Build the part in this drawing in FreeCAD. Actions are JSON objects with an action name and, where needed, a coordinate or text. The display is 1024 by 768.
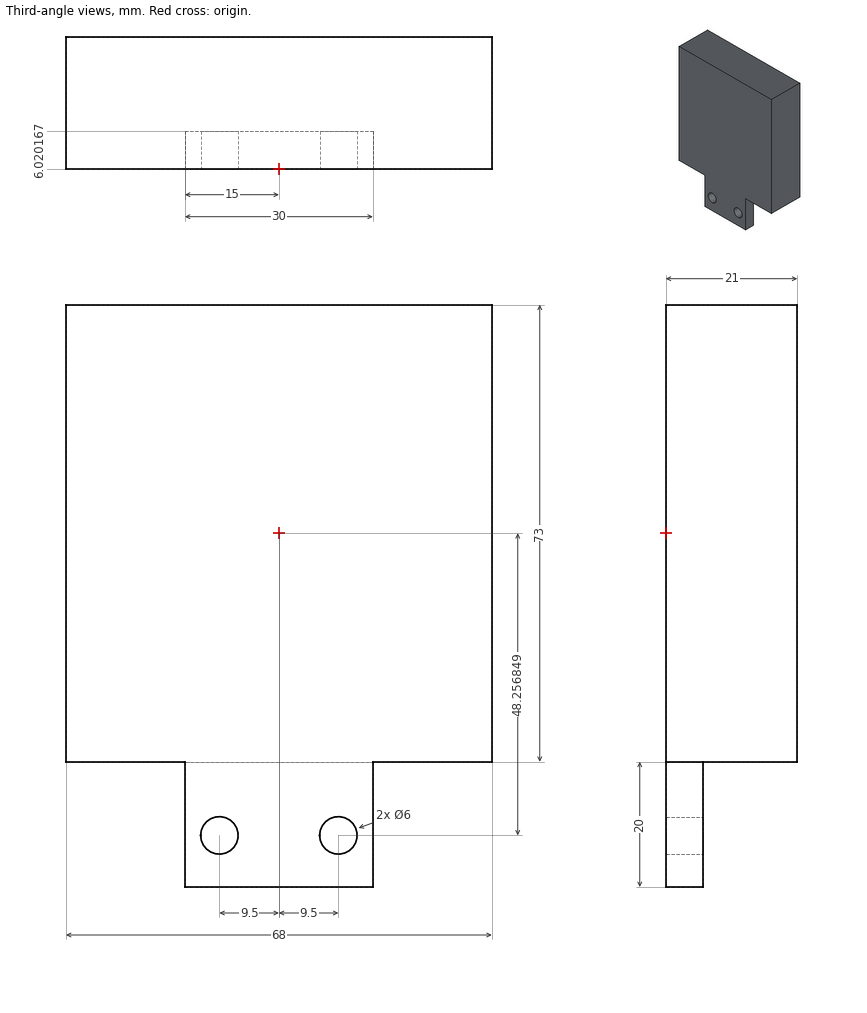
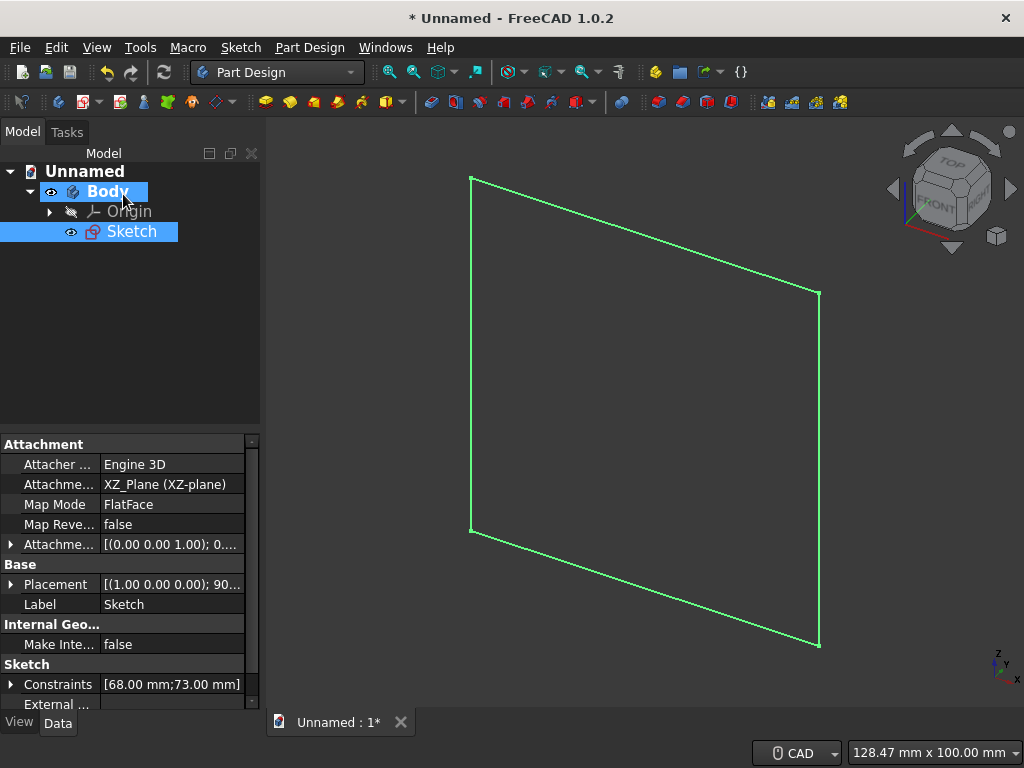
{"action": "left_click", "coordinate": [266, 102]}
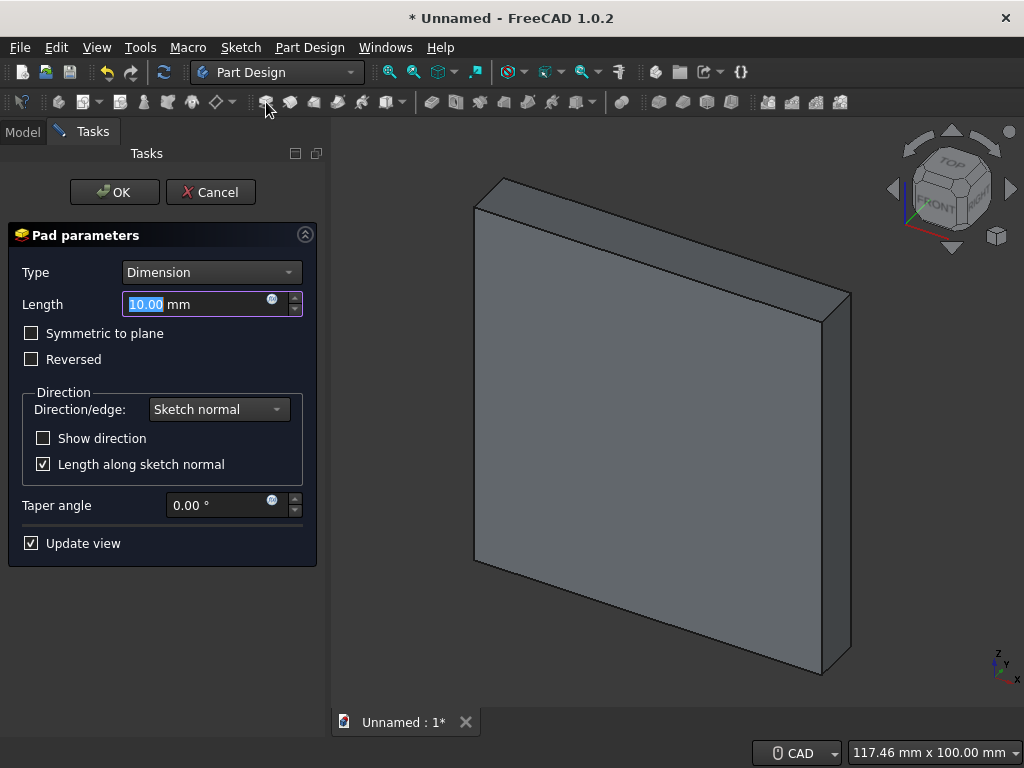
{"action": "type", "text": "21"}
{"action": "key", "text": "Tab"}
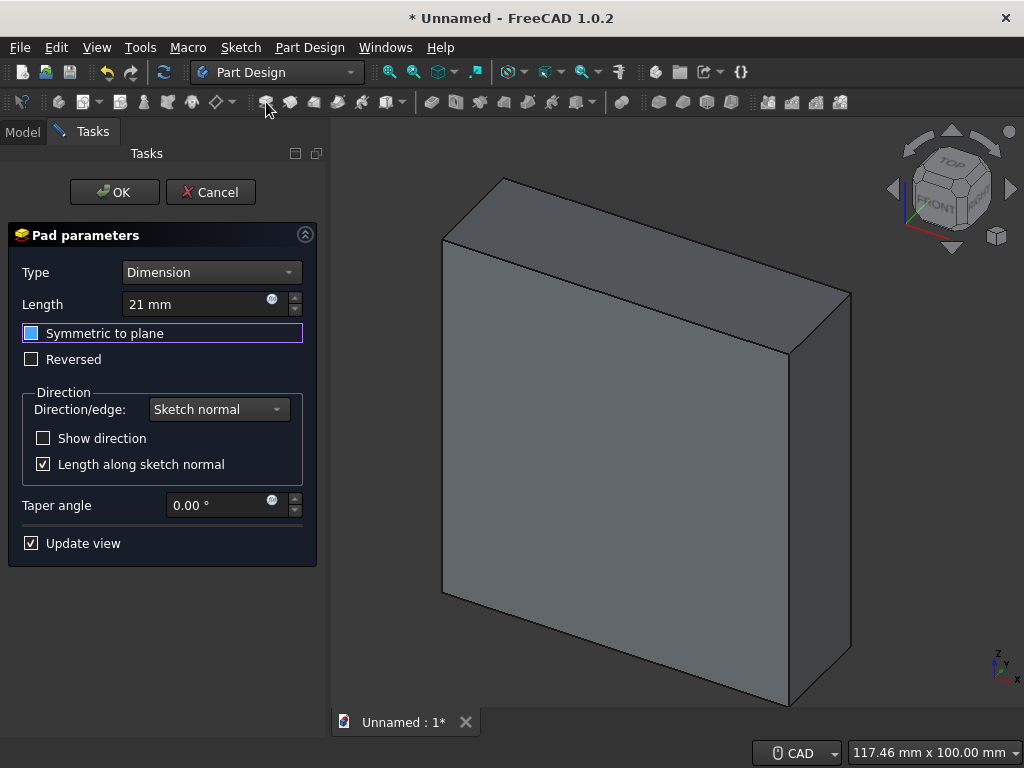
{"action": "left_click", "coordinate": [30, 359]}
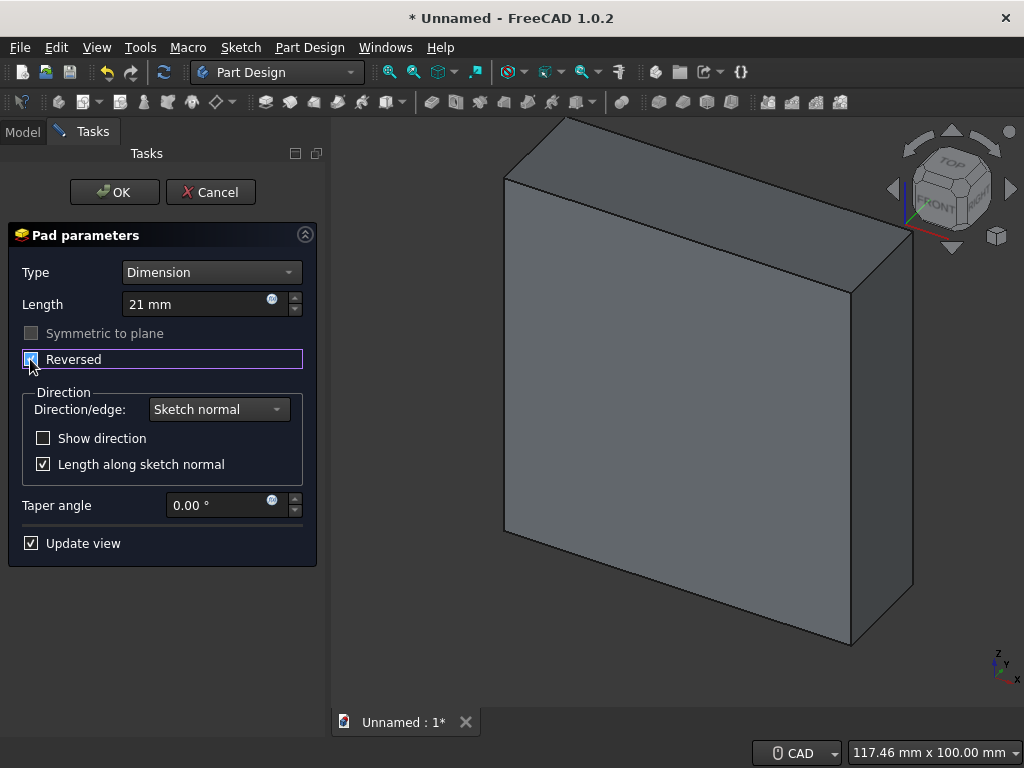
{"action": "left_click", "coordinate": [115, 192]}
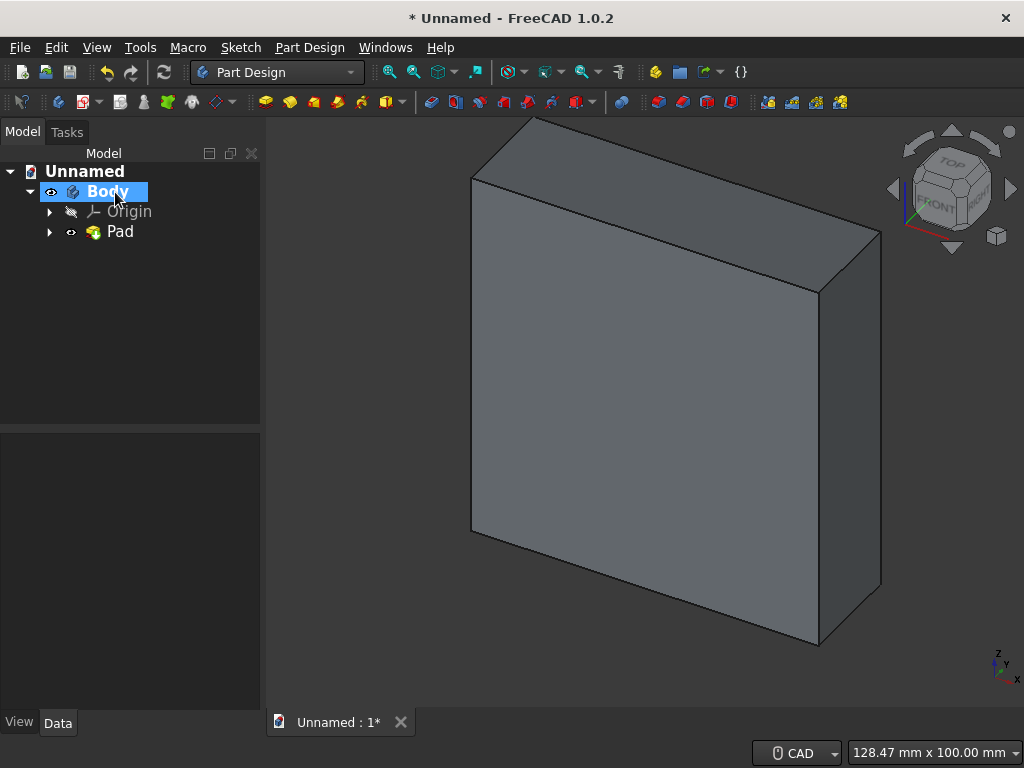
{"action": "key", "text": "v f"}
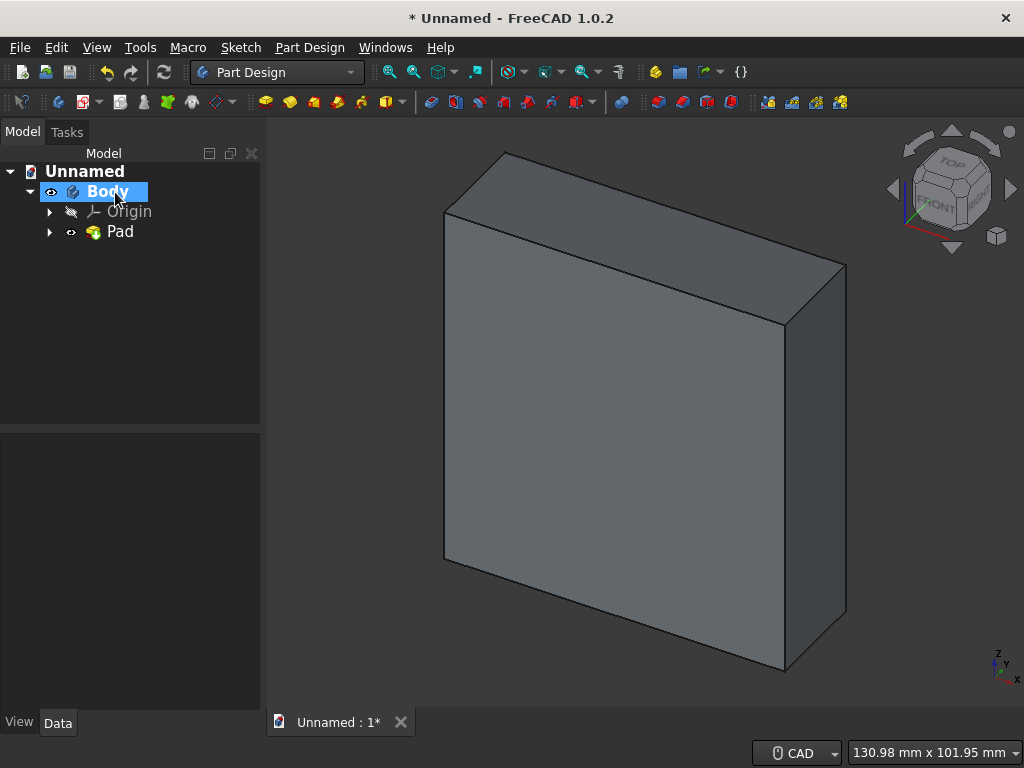
{"action": "key", "text": "5"}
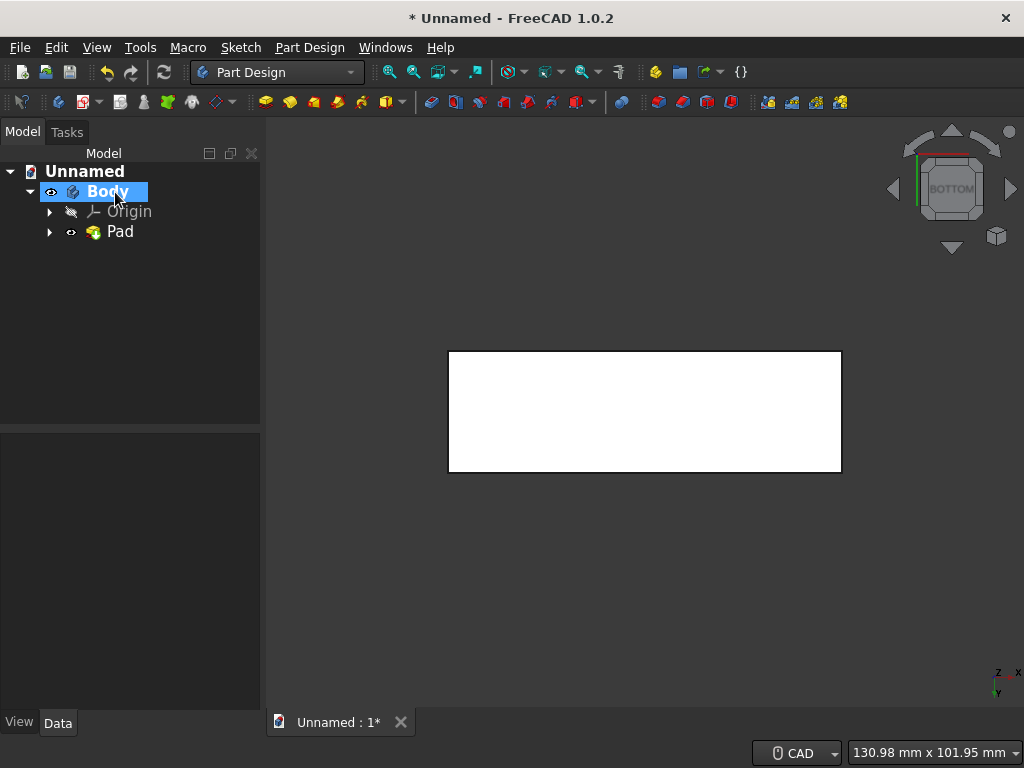
{"action": "left_click", "coordinate": [757, 411]}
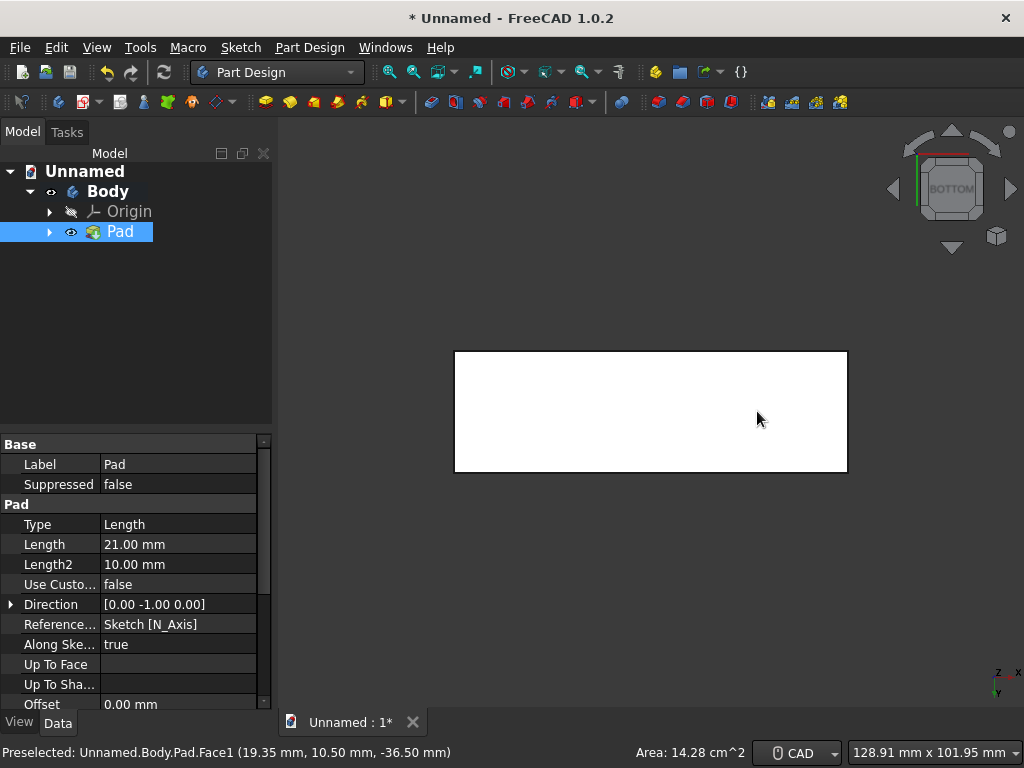
{"action": "left_click", "coordinate": [84, 102]}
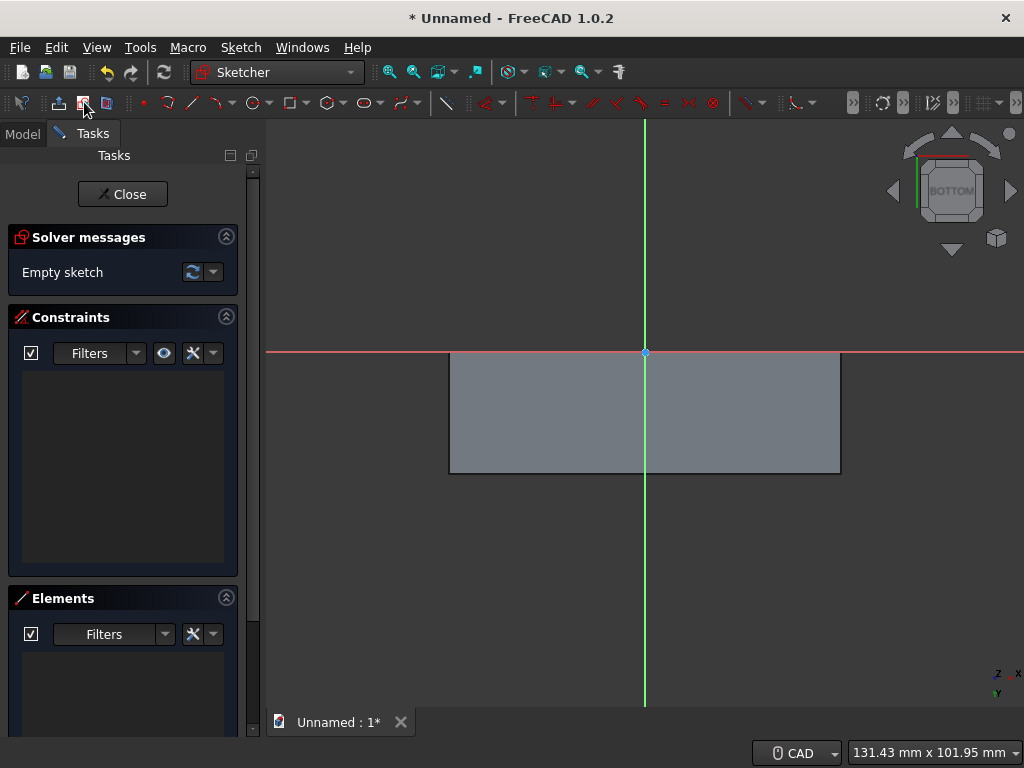
{"action": "scroll", "coordinate": [701, 335], "scroll_direction": "up", "scroll_amount": 4}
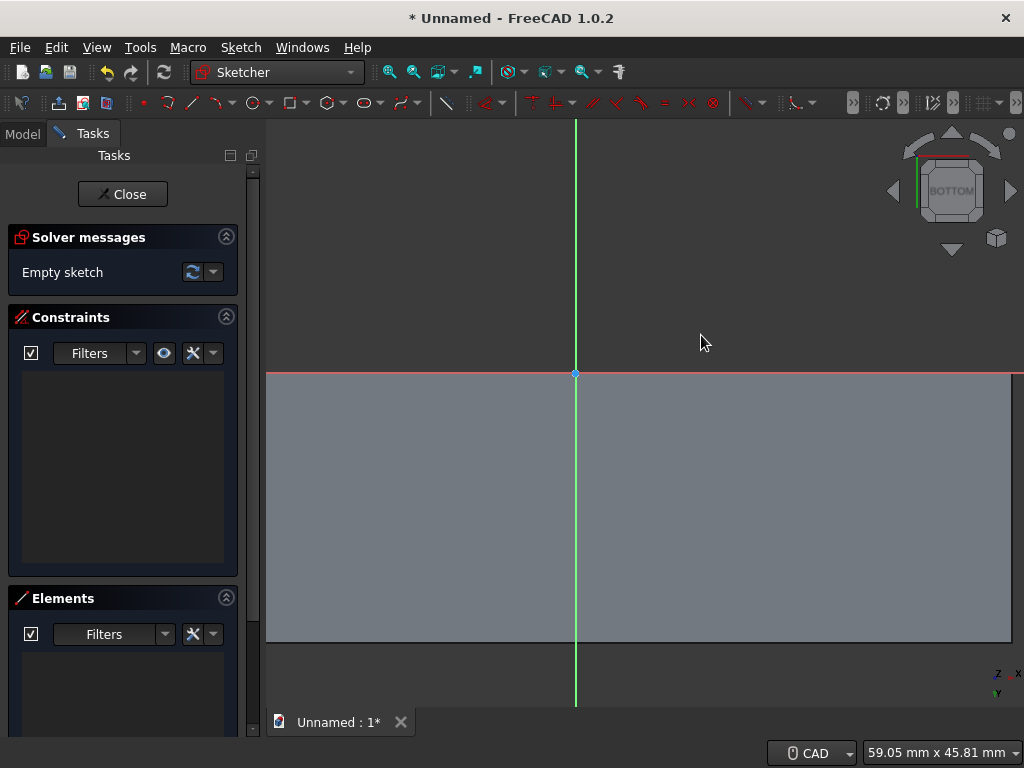
{"action": "key", "text": "g r"}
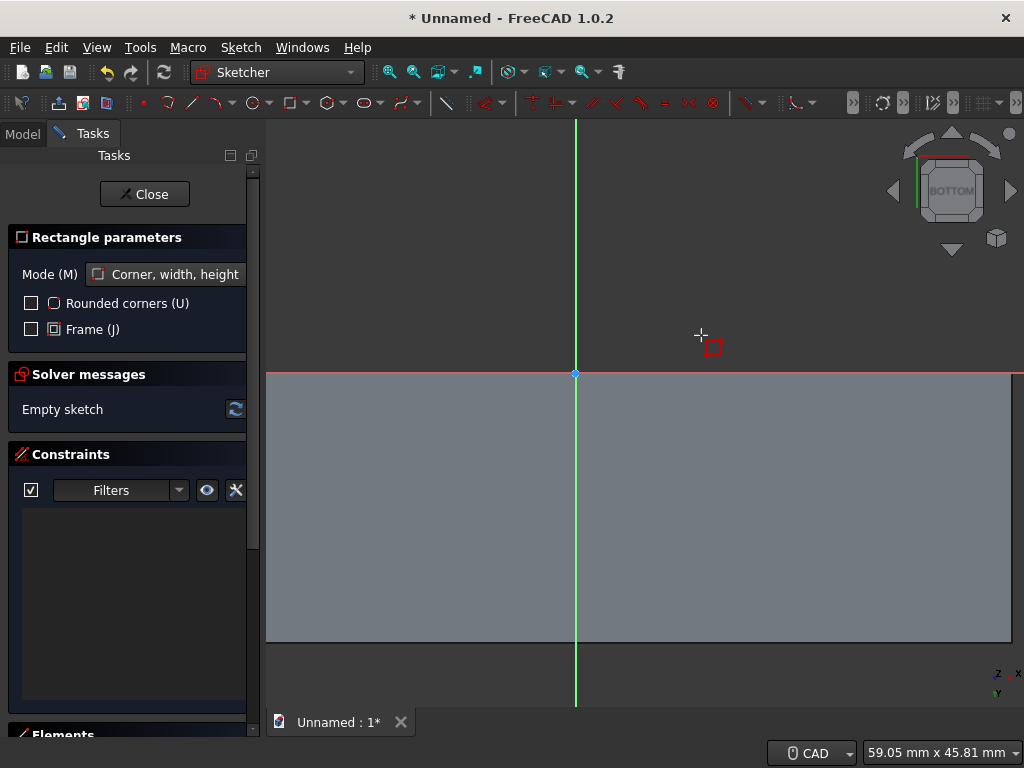
{"action": "left_click", "coordinate": [383, 373]}
{"action": "left_click", "coordinate": [768, 451]}
{"action": "key", "text": "Escape"}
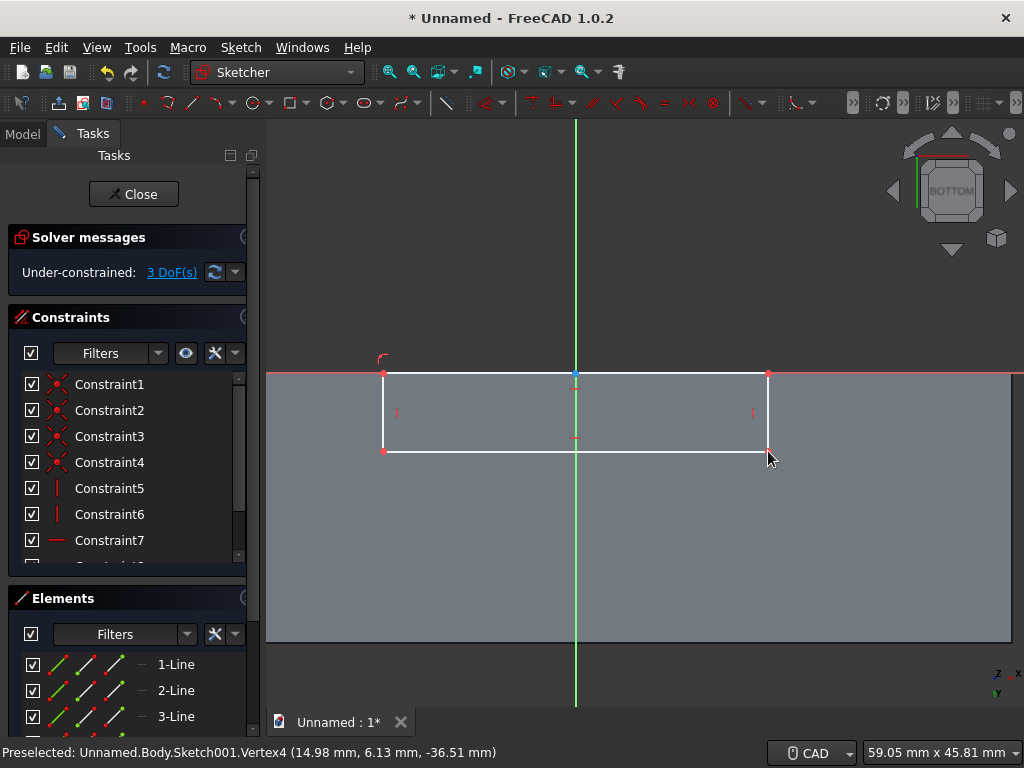
{"action": "left_click", "coordinate": [486, 104]}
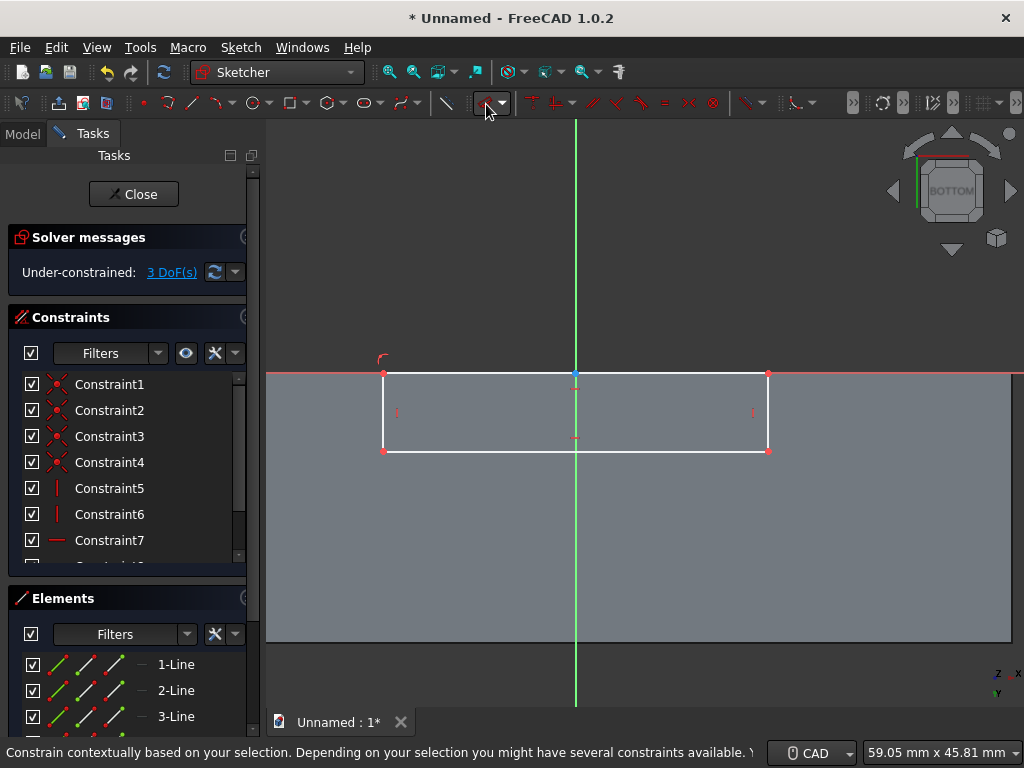
{"action": "left_click", "coordinate": [499, 452]}
{"action": "left_click", "coordinate": [487, 486]}